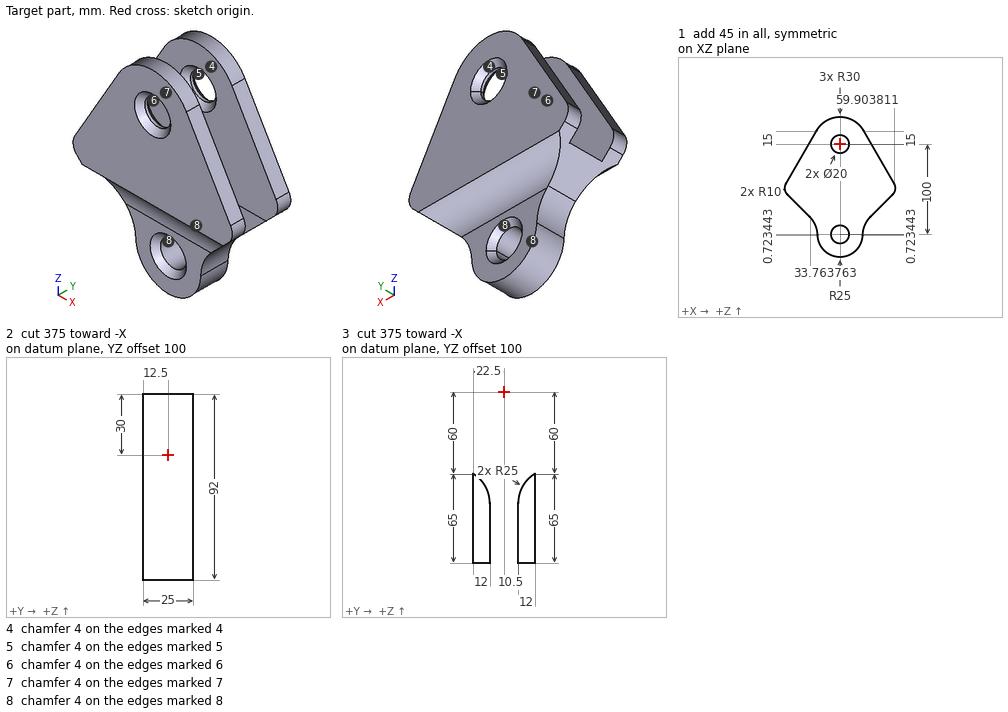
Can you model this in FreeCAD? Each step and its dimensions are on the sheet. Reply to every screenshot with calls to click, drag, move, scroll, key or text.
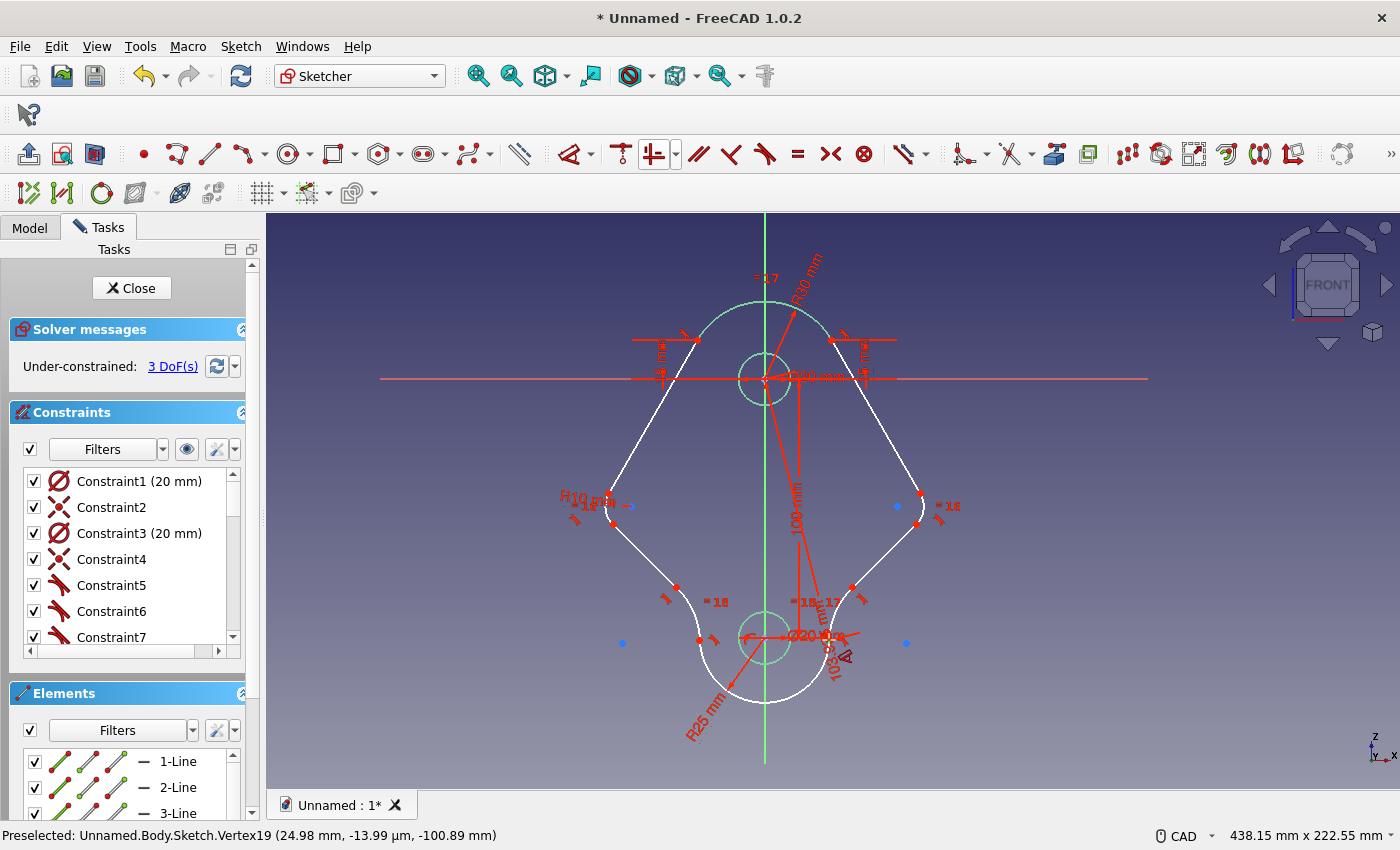
scroll(765, 638, up, 16)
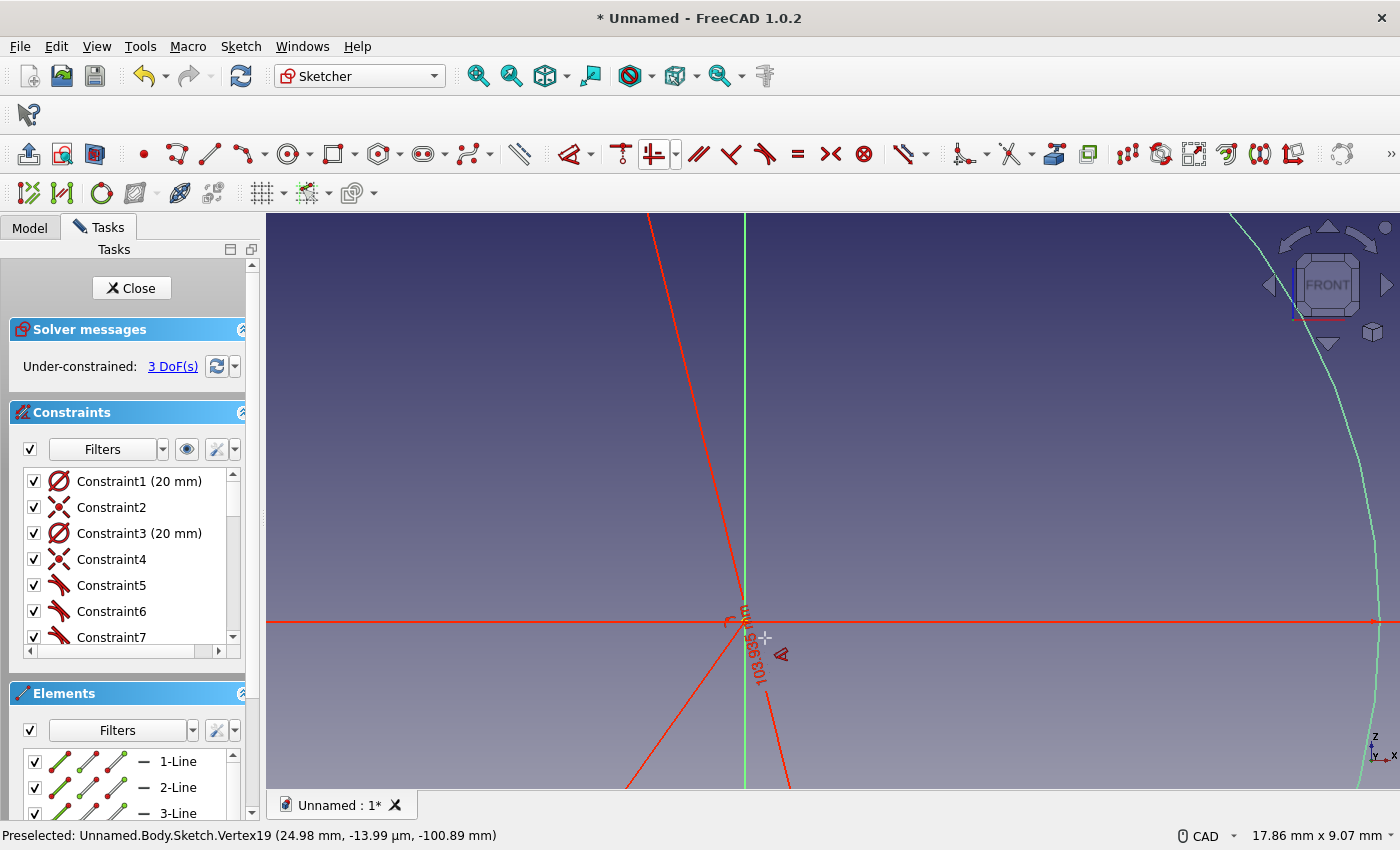
click(745, 622)
click(711, 650)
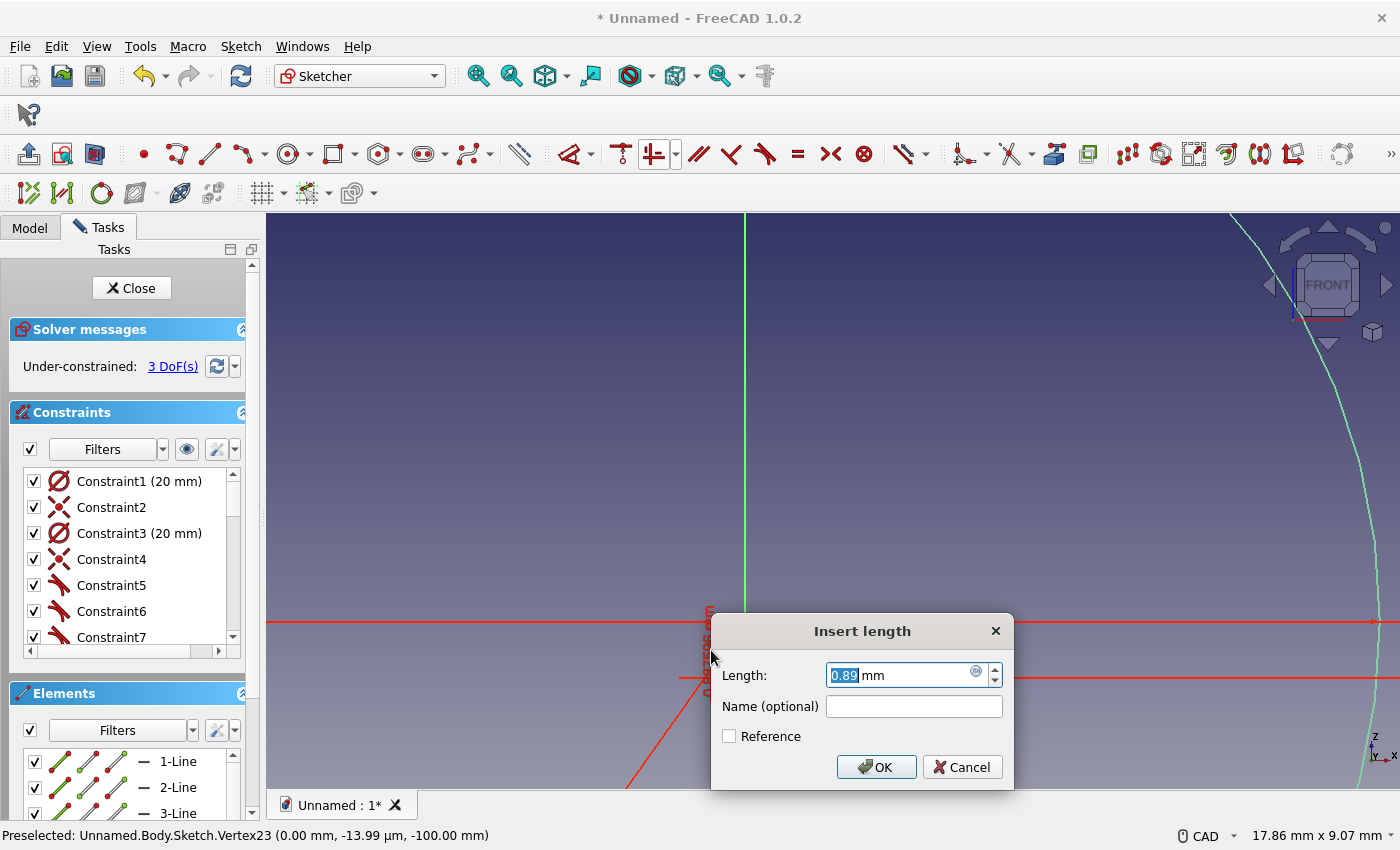
text(0.723443)
key(Return)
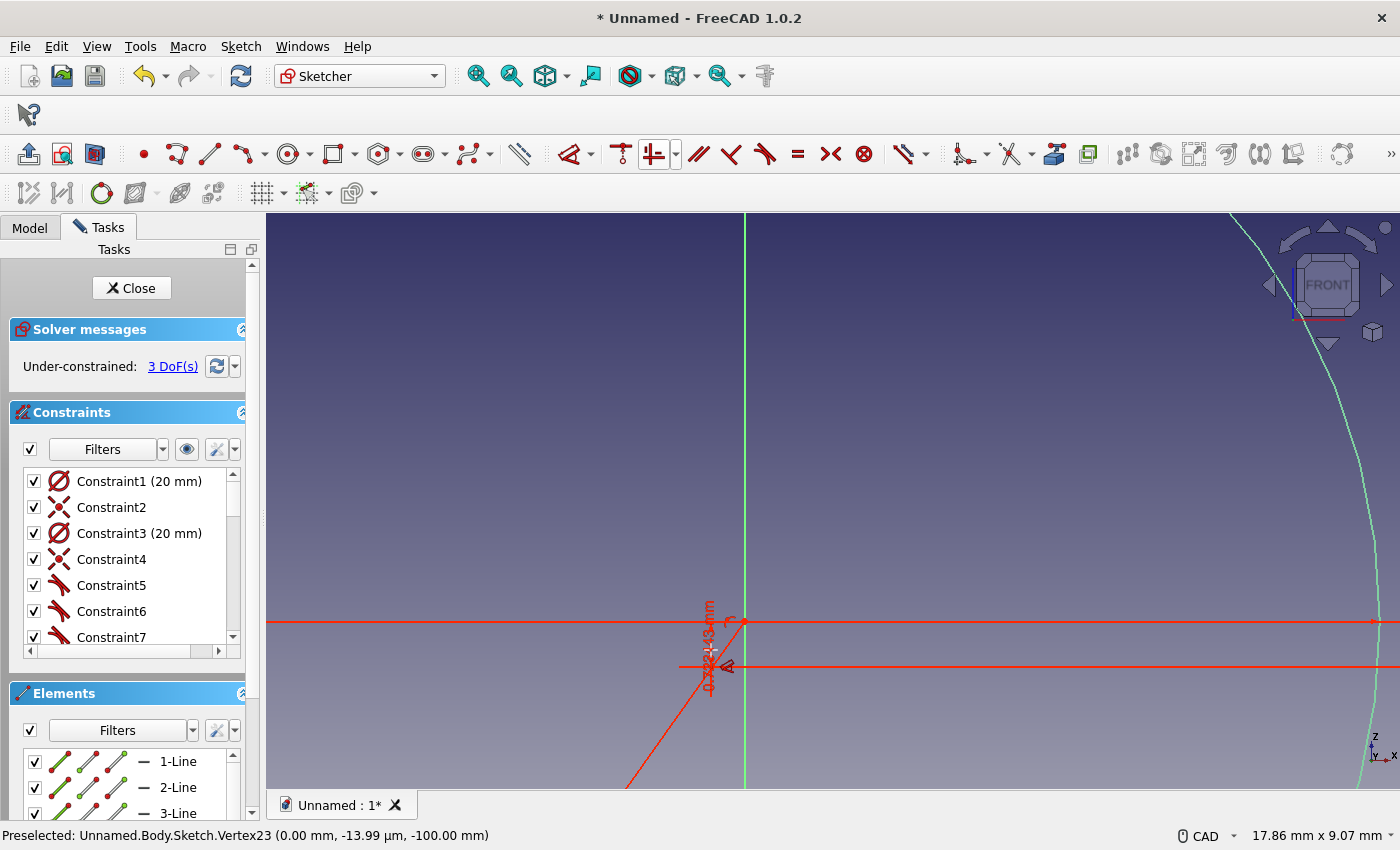
scroll(765, 638, down, 16)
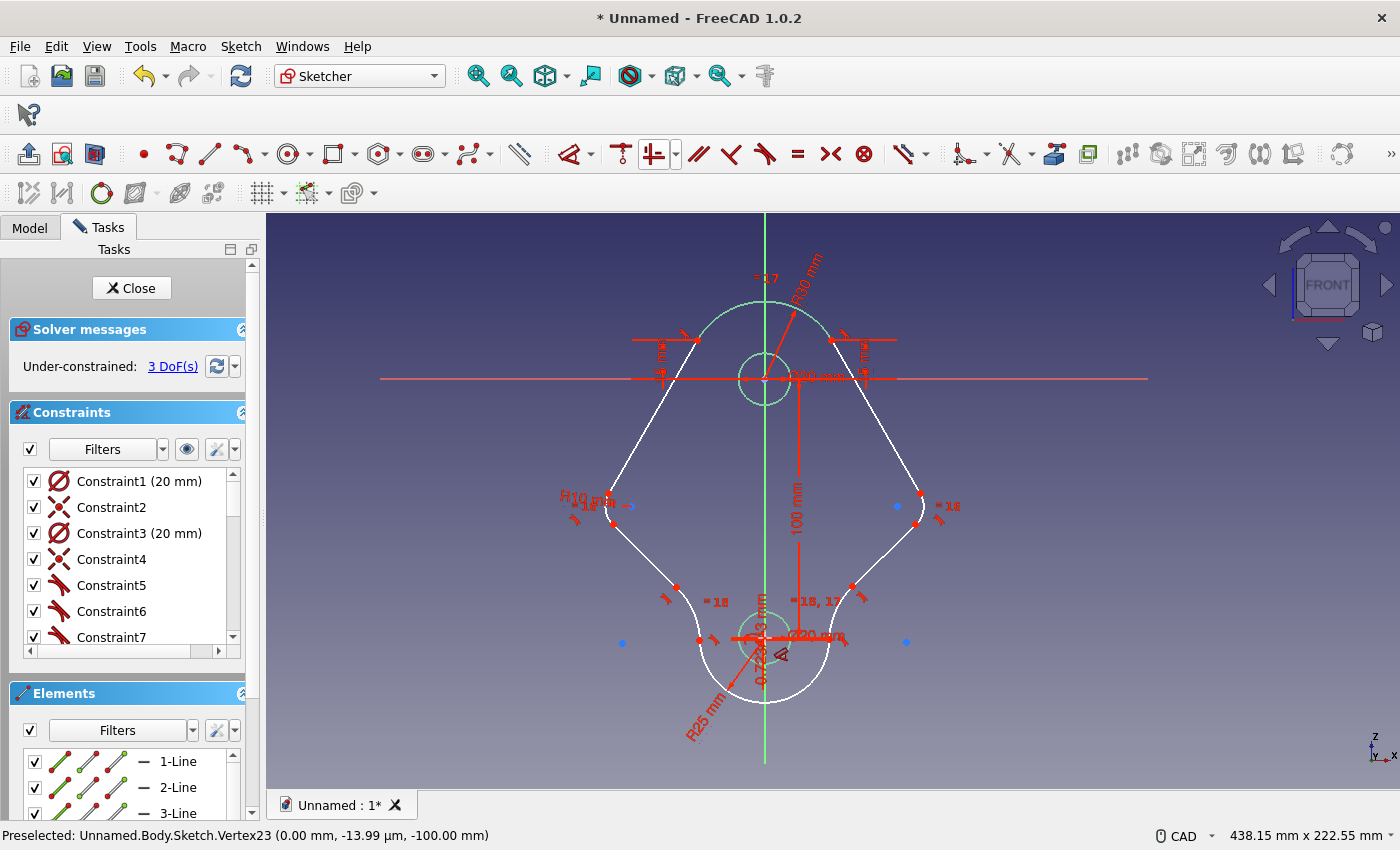
scroll(700, 640, up, 16)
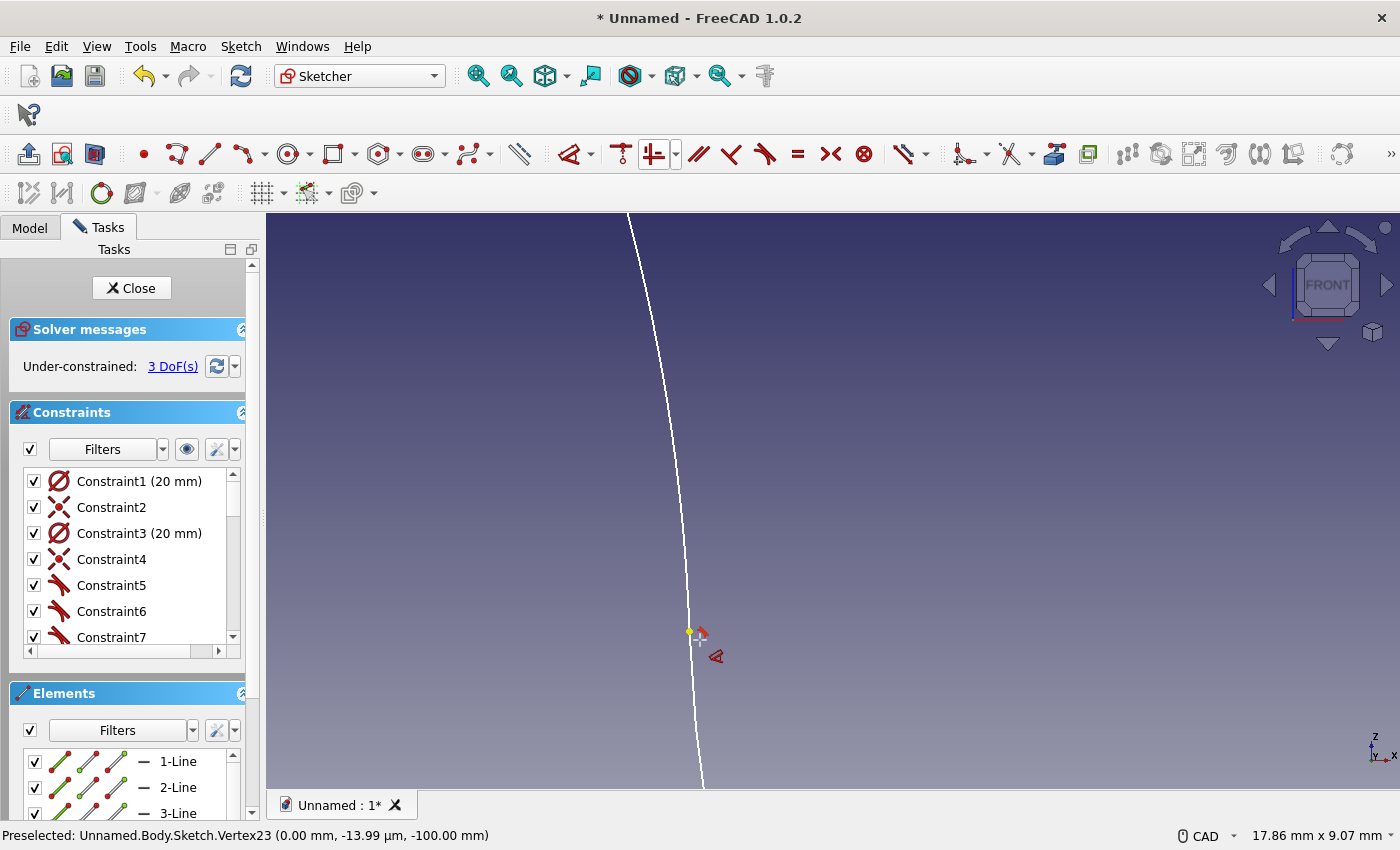
click(690, 632)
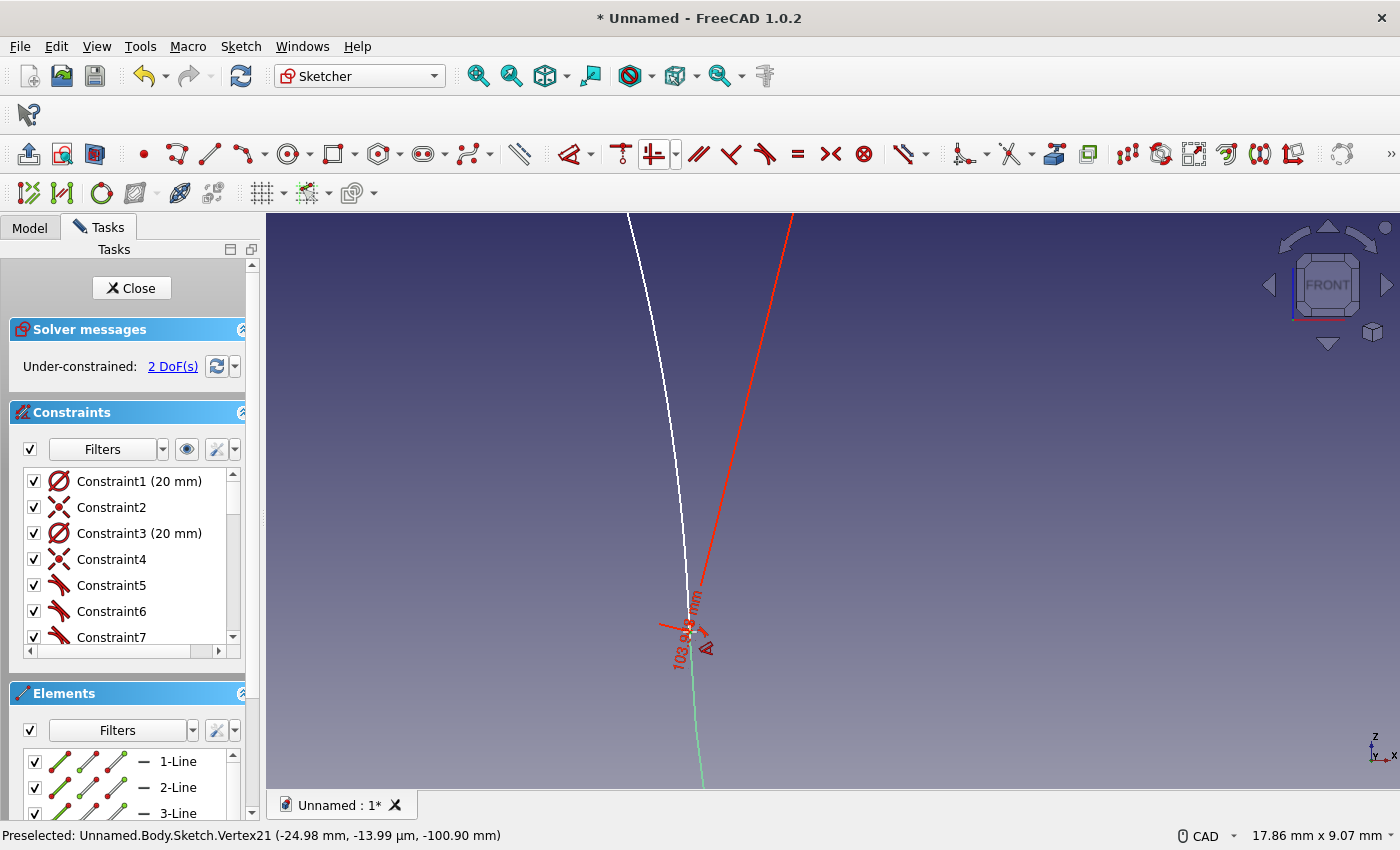
scroll(700, 640, down, 16)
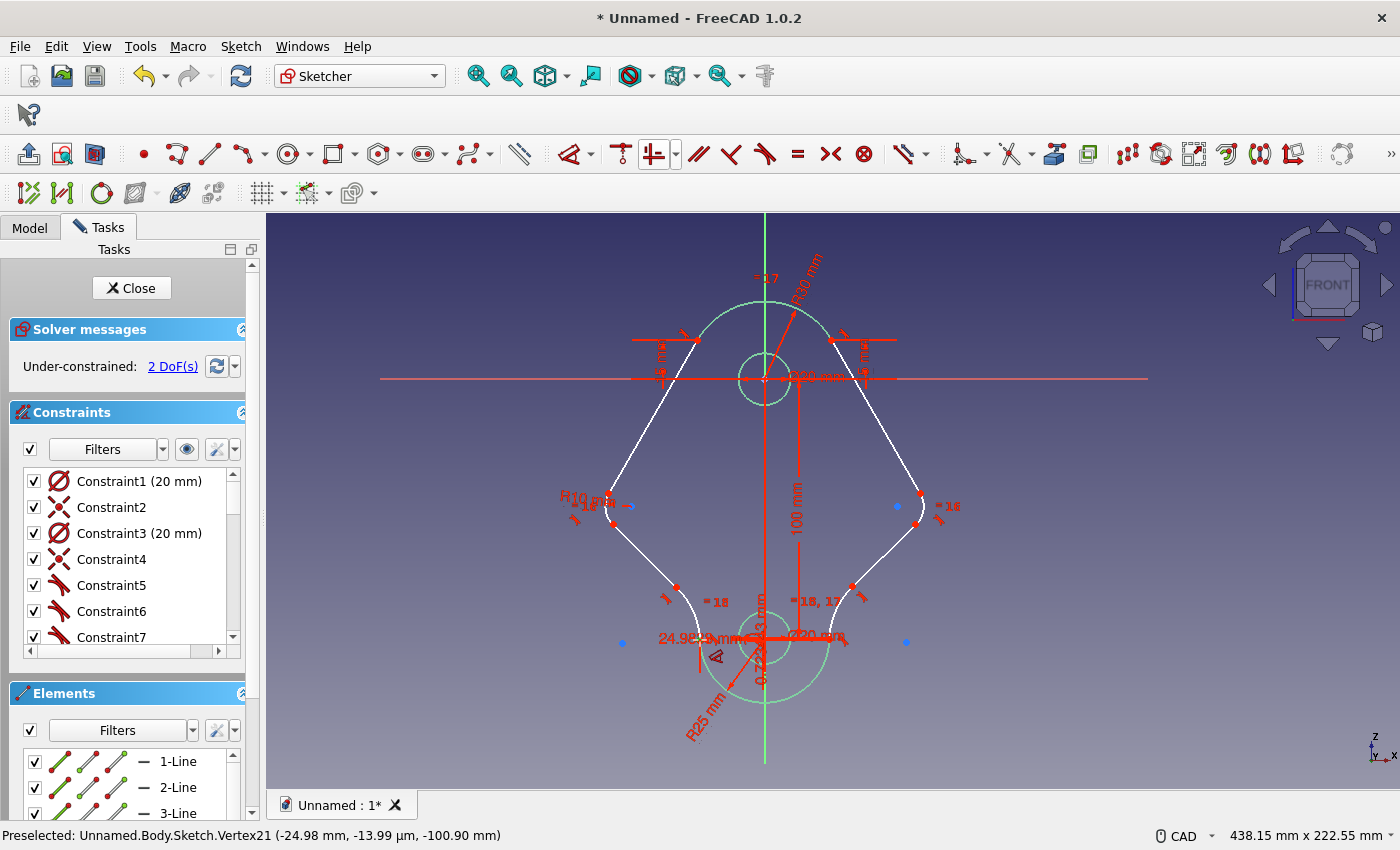
scroll(765, 638, up, 16)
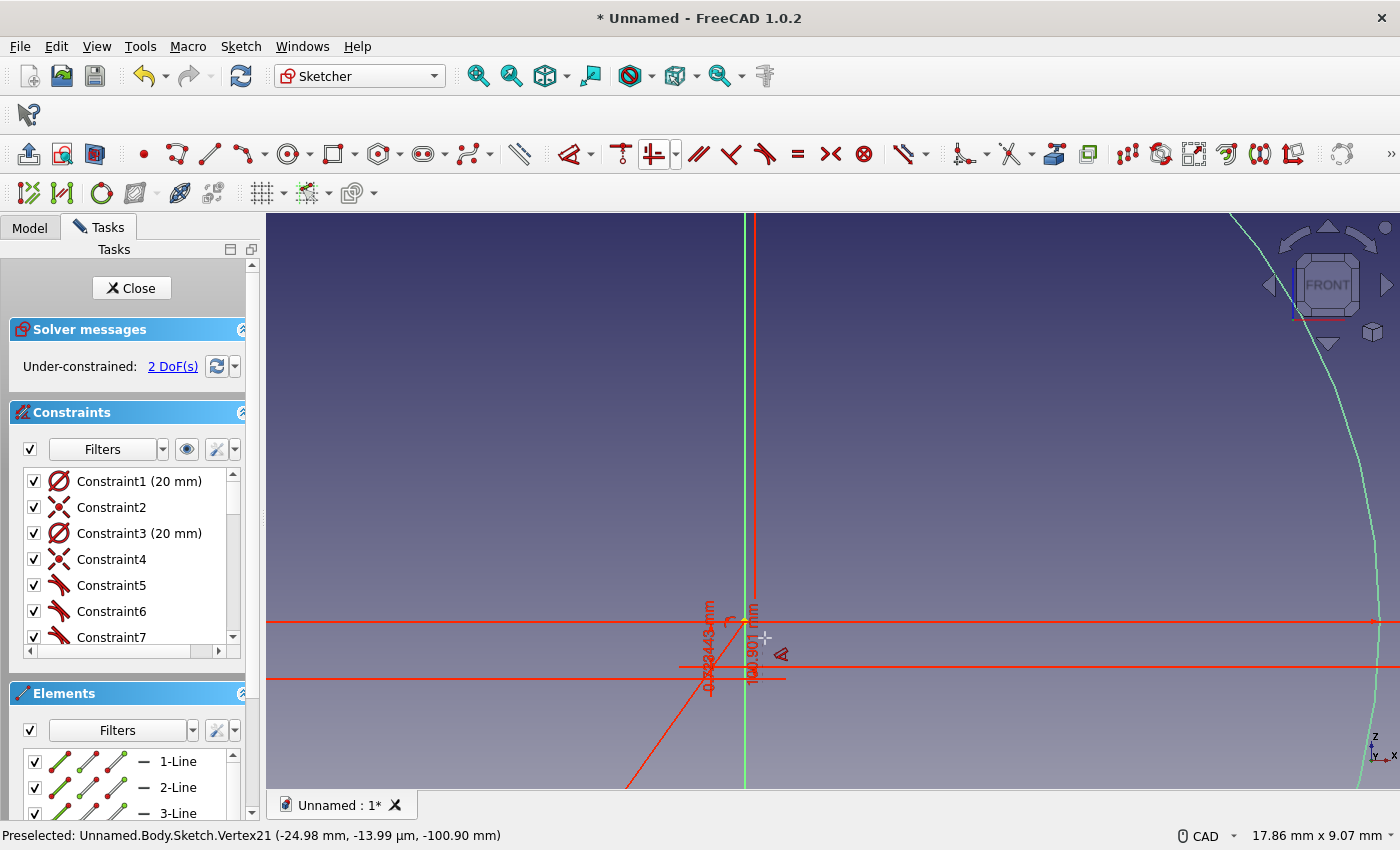
click(745, 622)
click(779, 670)